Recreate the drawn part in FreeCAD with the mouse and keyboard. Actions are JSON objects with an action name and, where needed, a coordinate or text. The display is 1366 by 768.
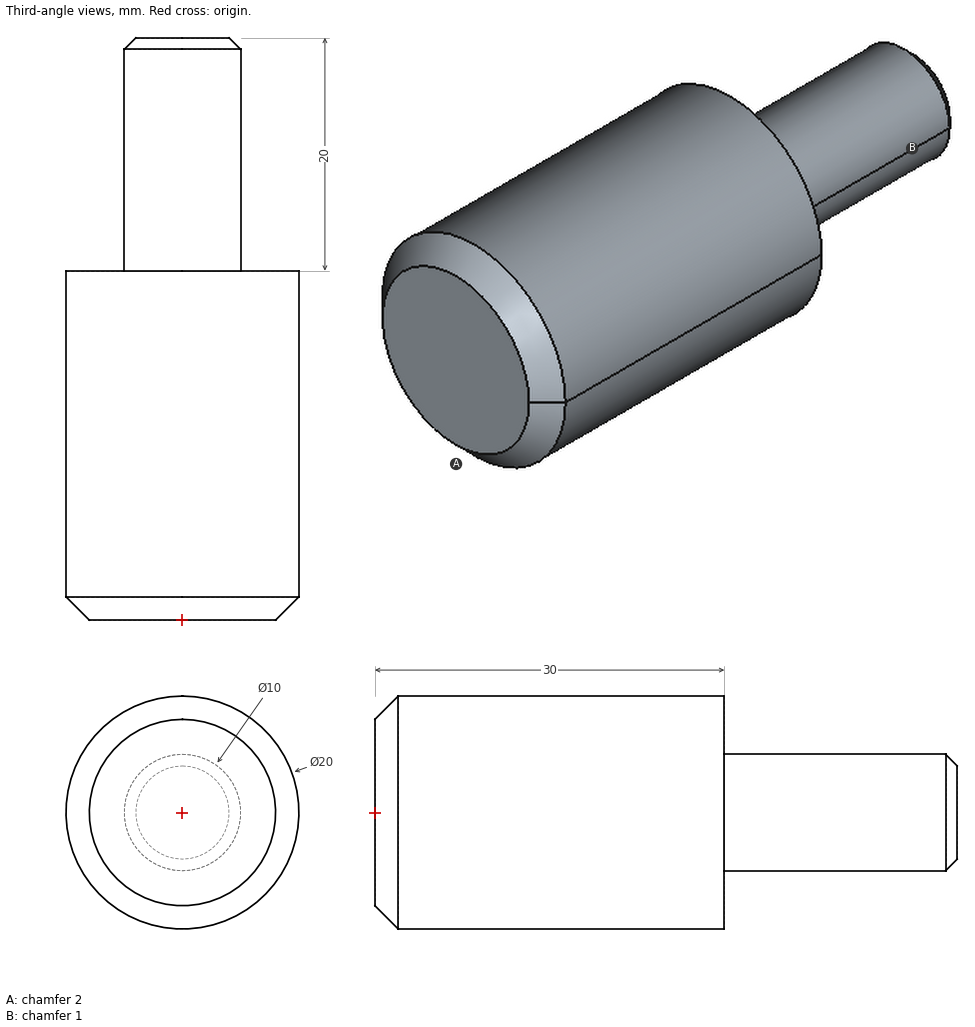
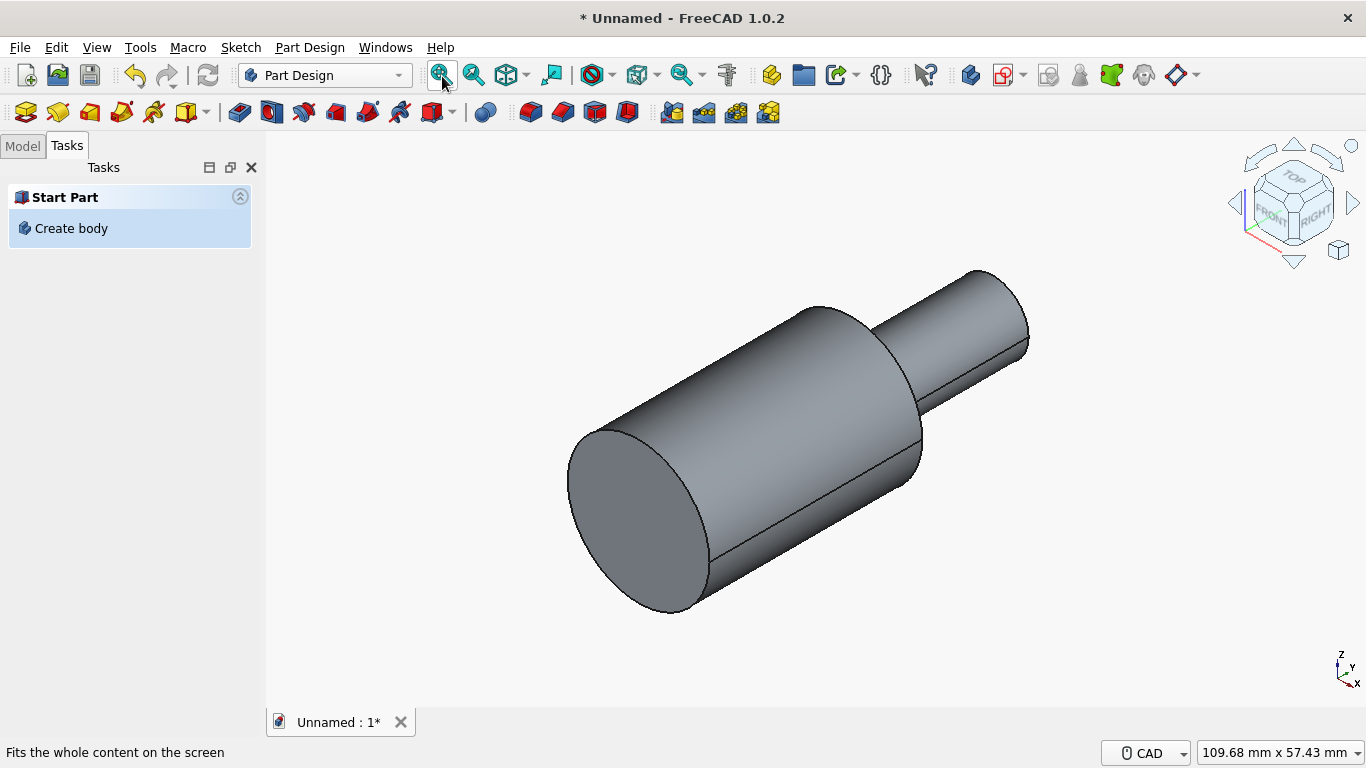
{"action": "left_click", "coordinate": [617, 430]}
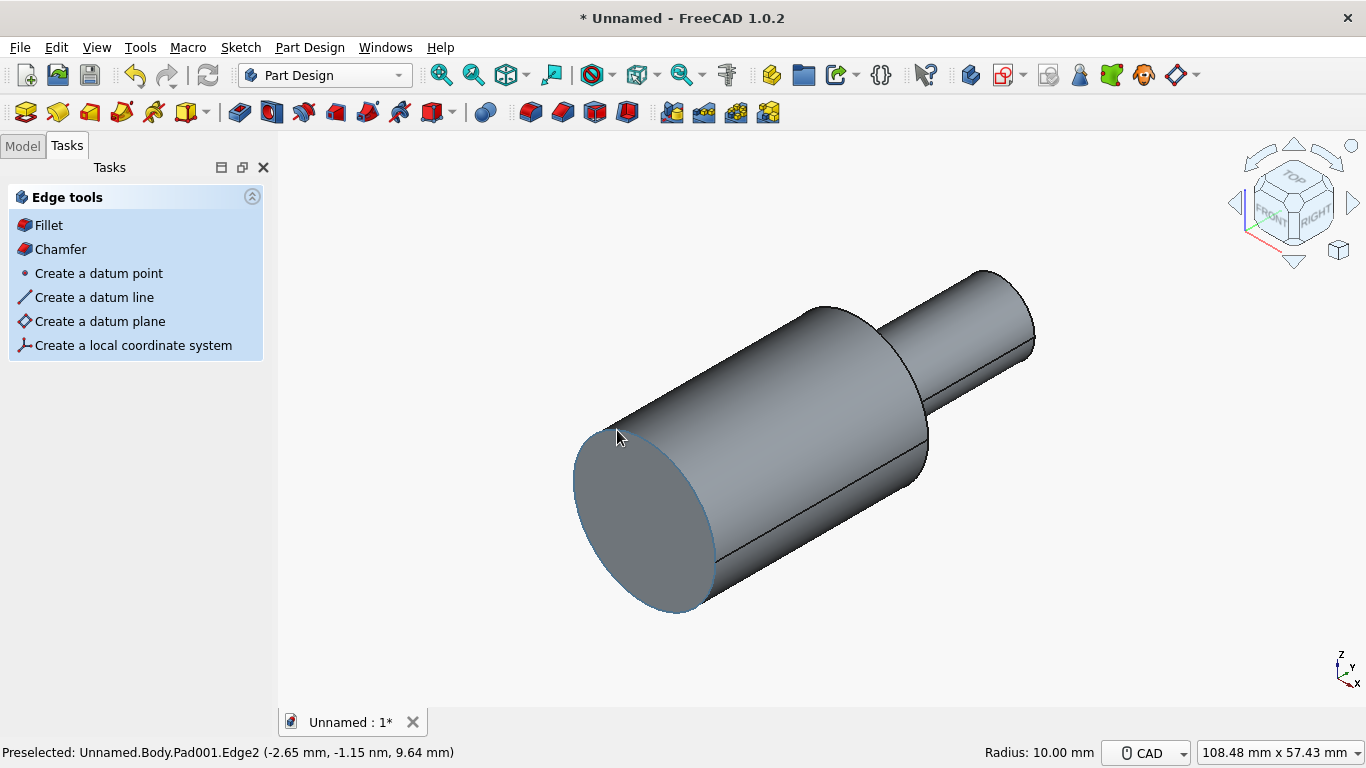
{"action": "left_click", "coordinate": [564, 112]}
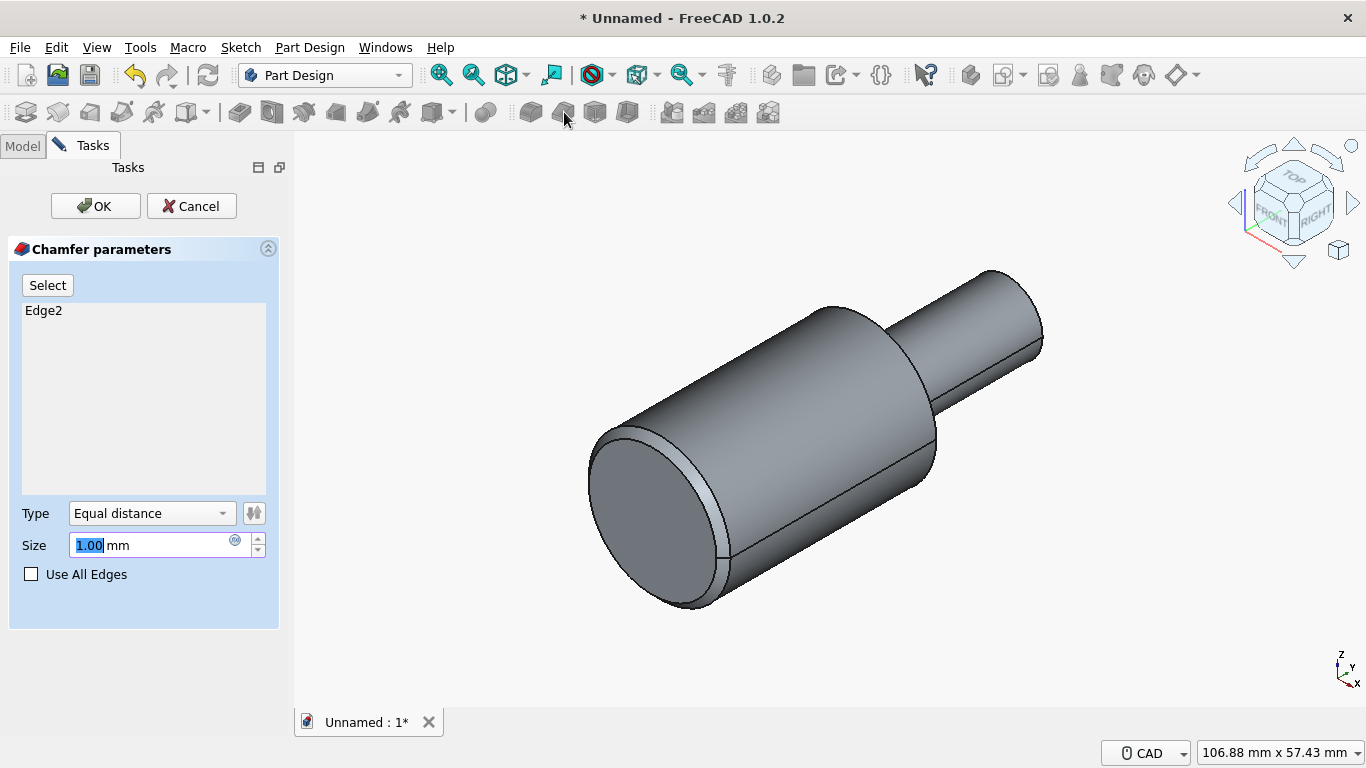
{"action": "type", "text": "2"}
{"action": "key", "text": "Tab"}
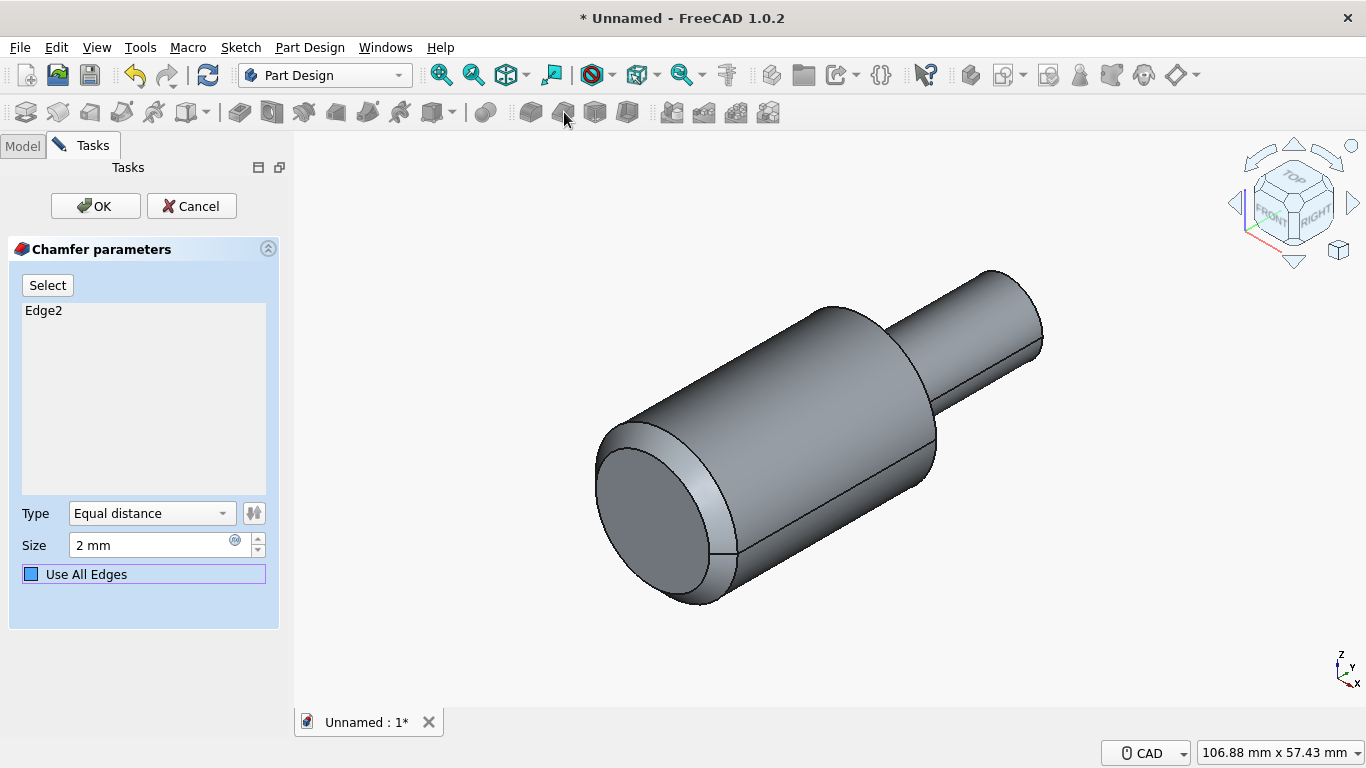
{"action": "left_click", "coordinate": [96, 206]}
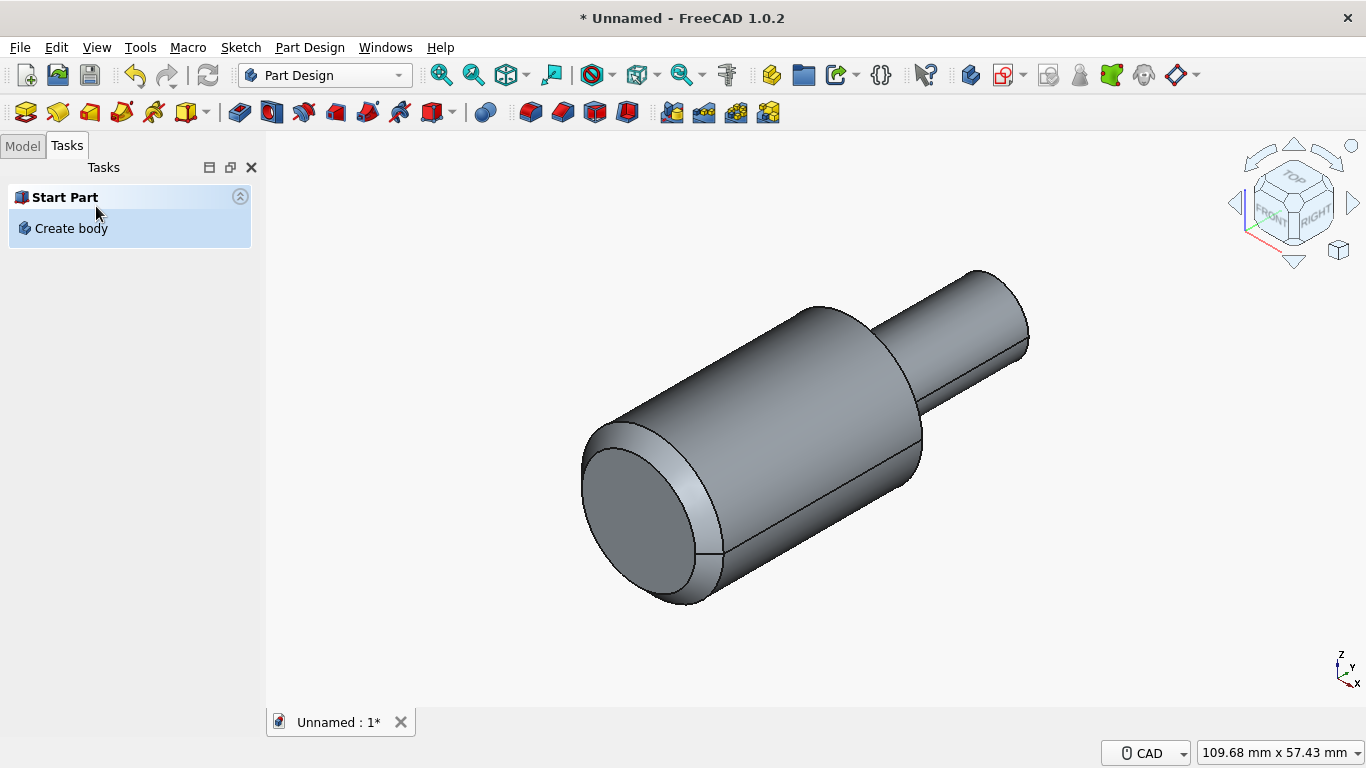
{"action": "key", "text": "2"}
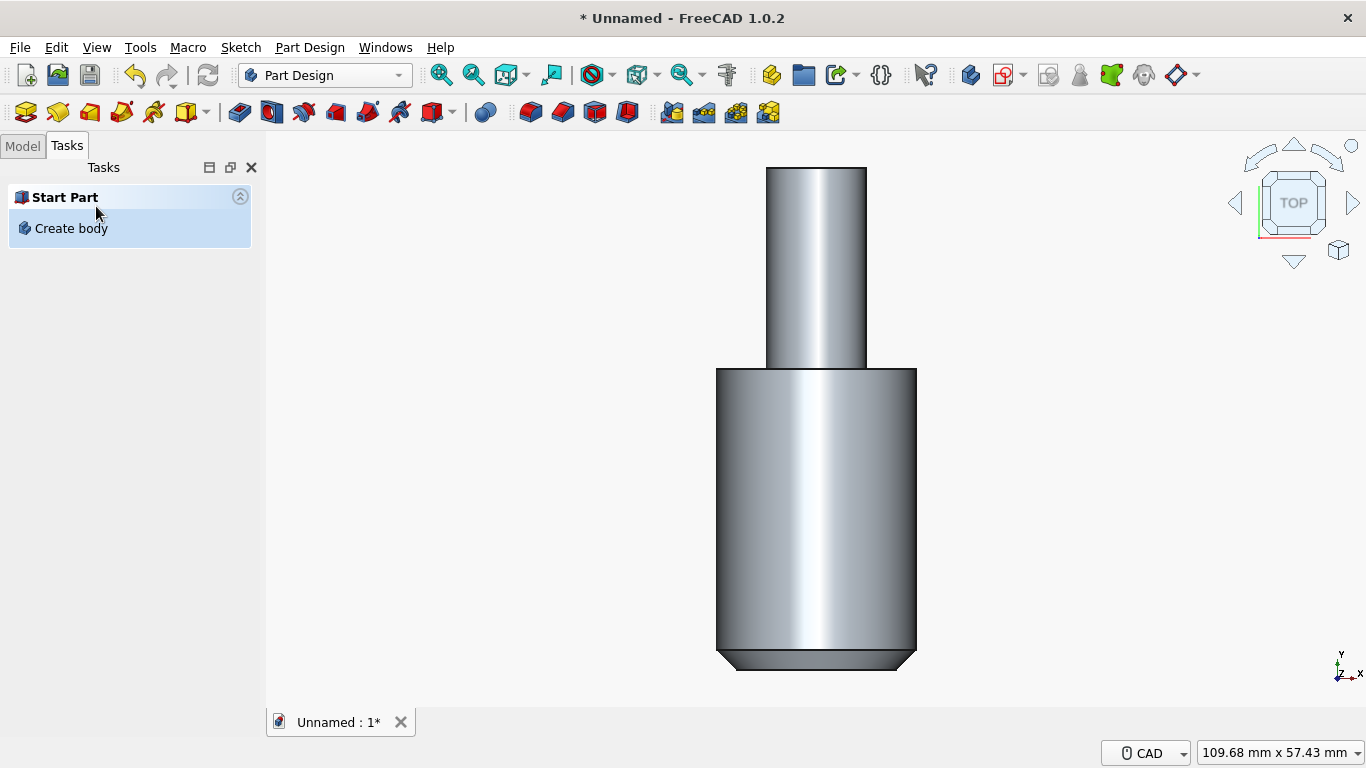
{"action": "left_click", "coordinate": [766, 167]}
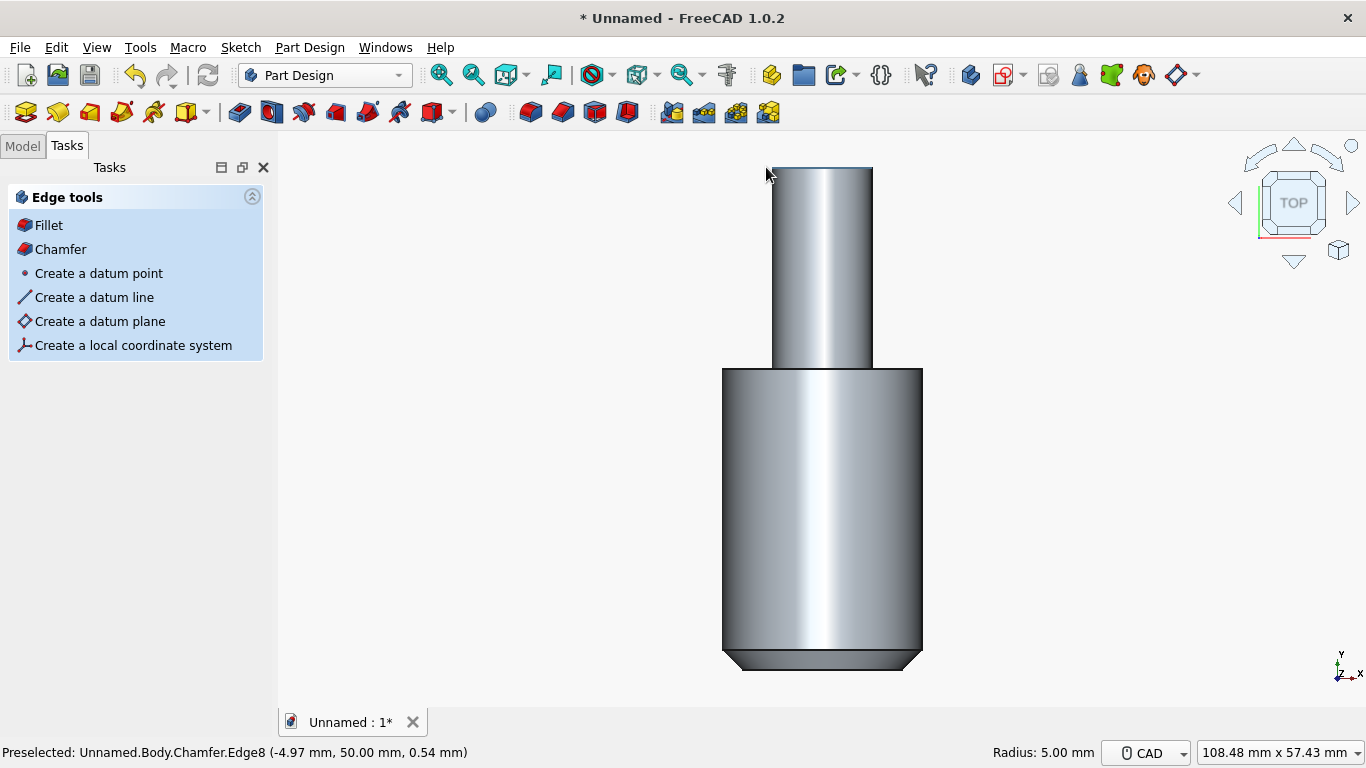
{"action": "left_click", "coordinate": [564, 112]}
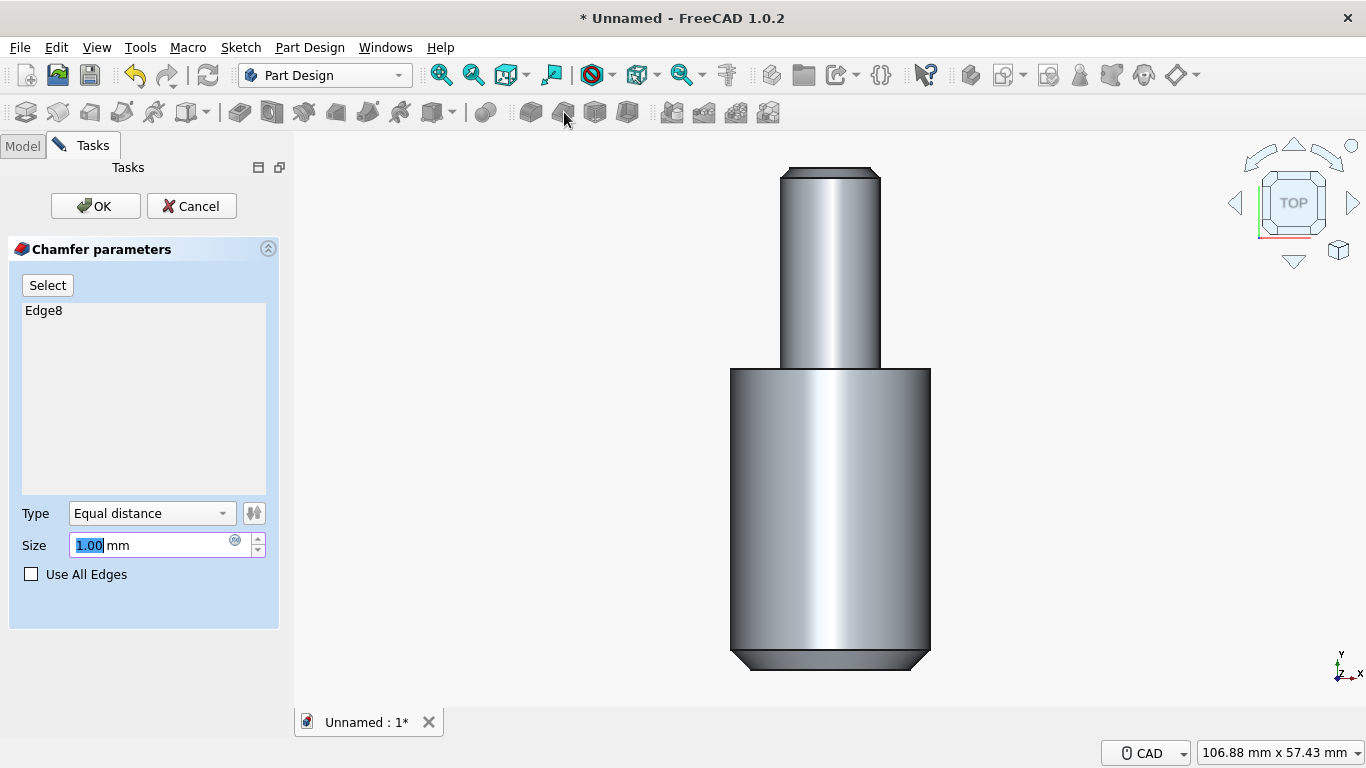
{"action": "type", "text": "1"}
{"action": "key", "text": "Tab"}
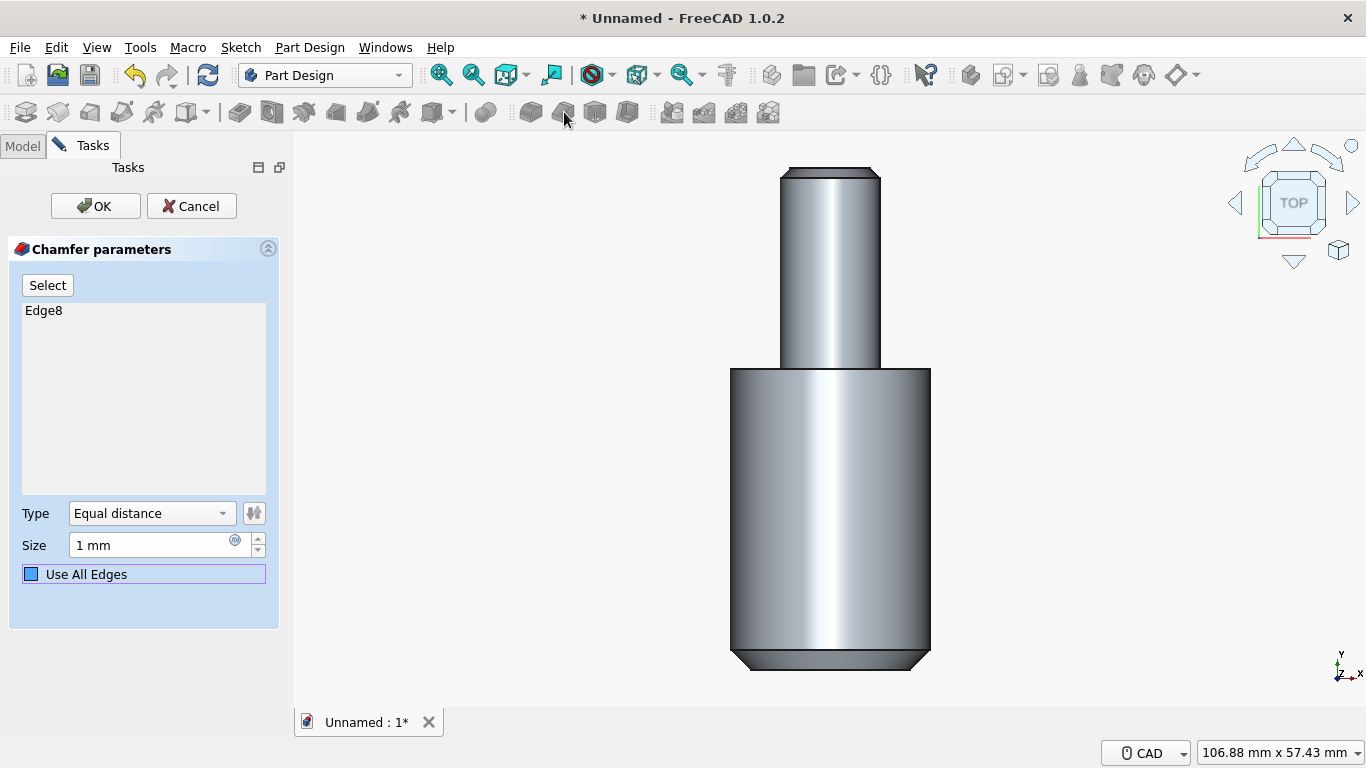
{"action": "left_click", "coordinate": [96, 206]}